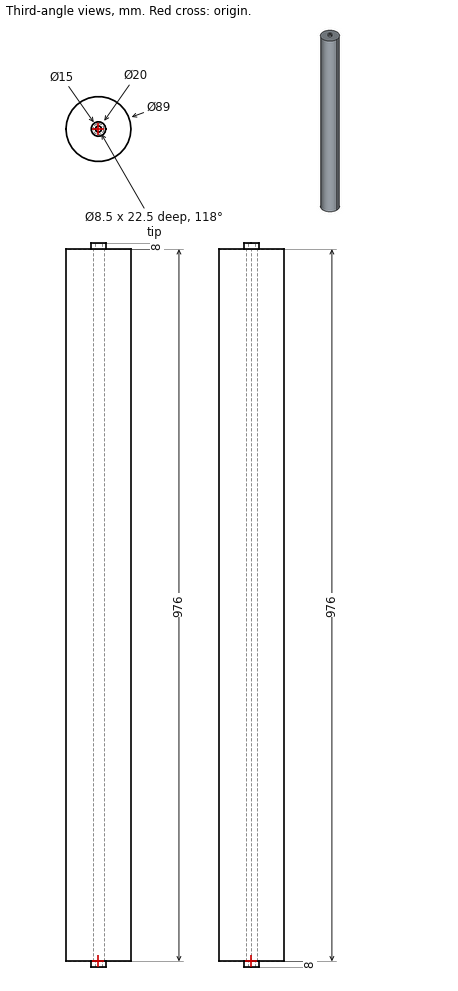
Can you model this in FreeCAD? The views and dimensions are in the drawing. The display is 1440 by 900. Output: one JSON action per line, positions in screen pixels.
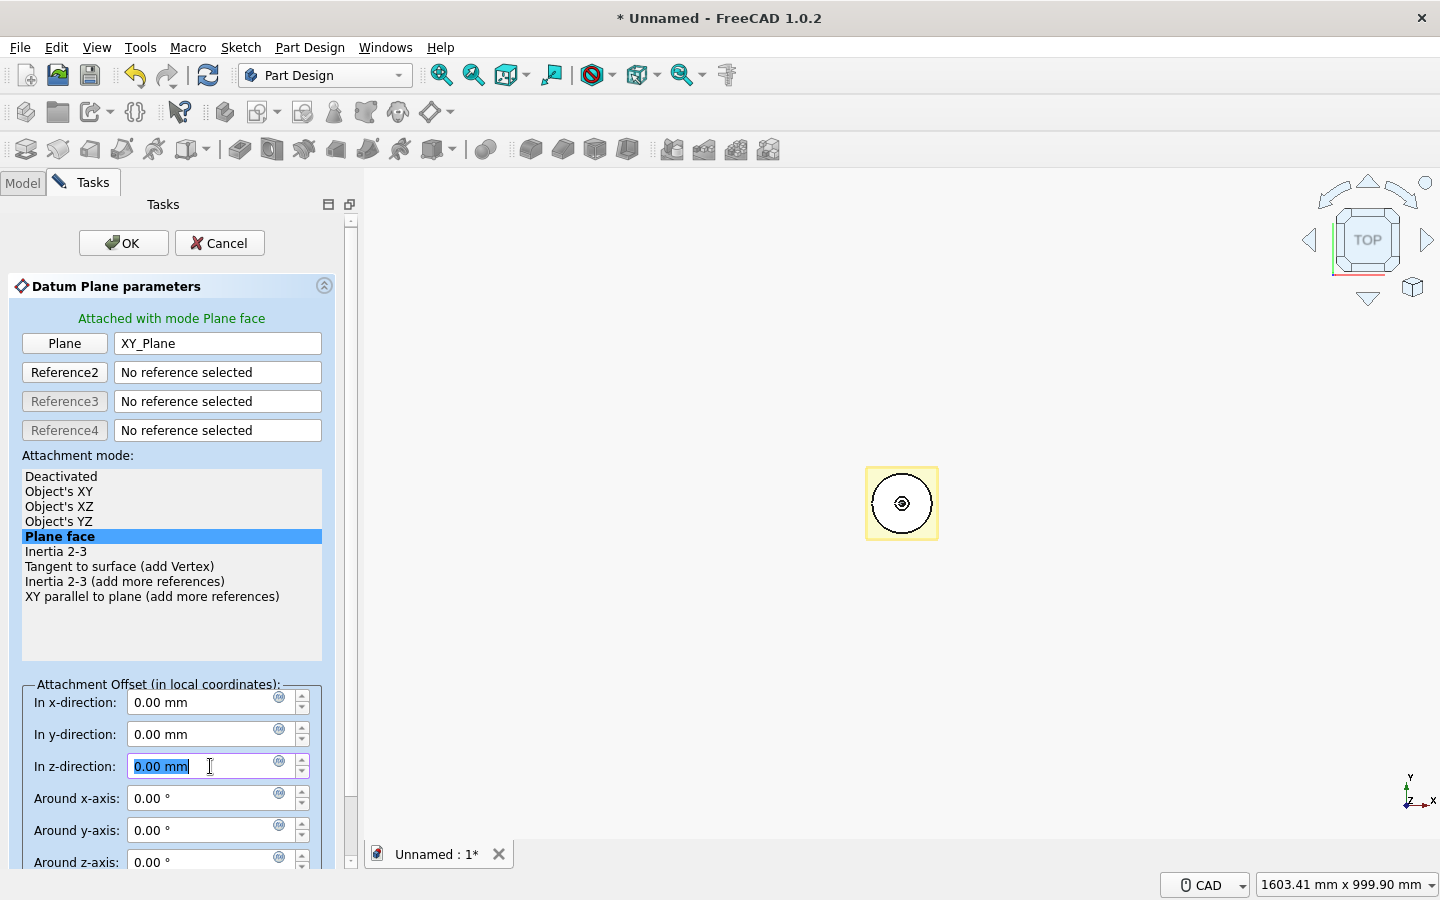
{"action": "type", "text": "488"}
{"action": "key", "text": "Tab"}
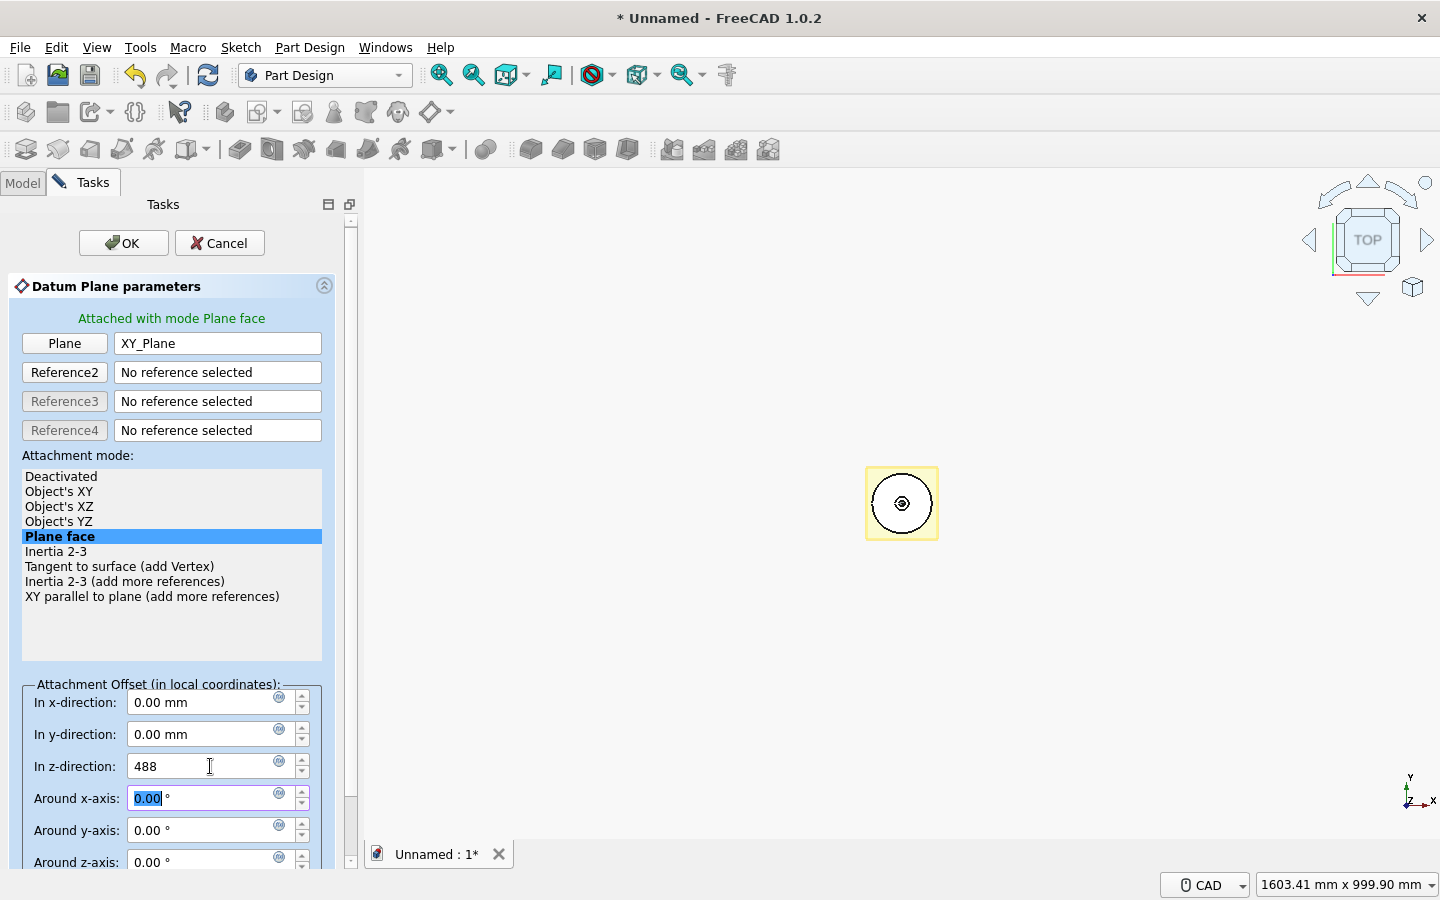
{"action": "left_click", "coordinate": [124, 243]}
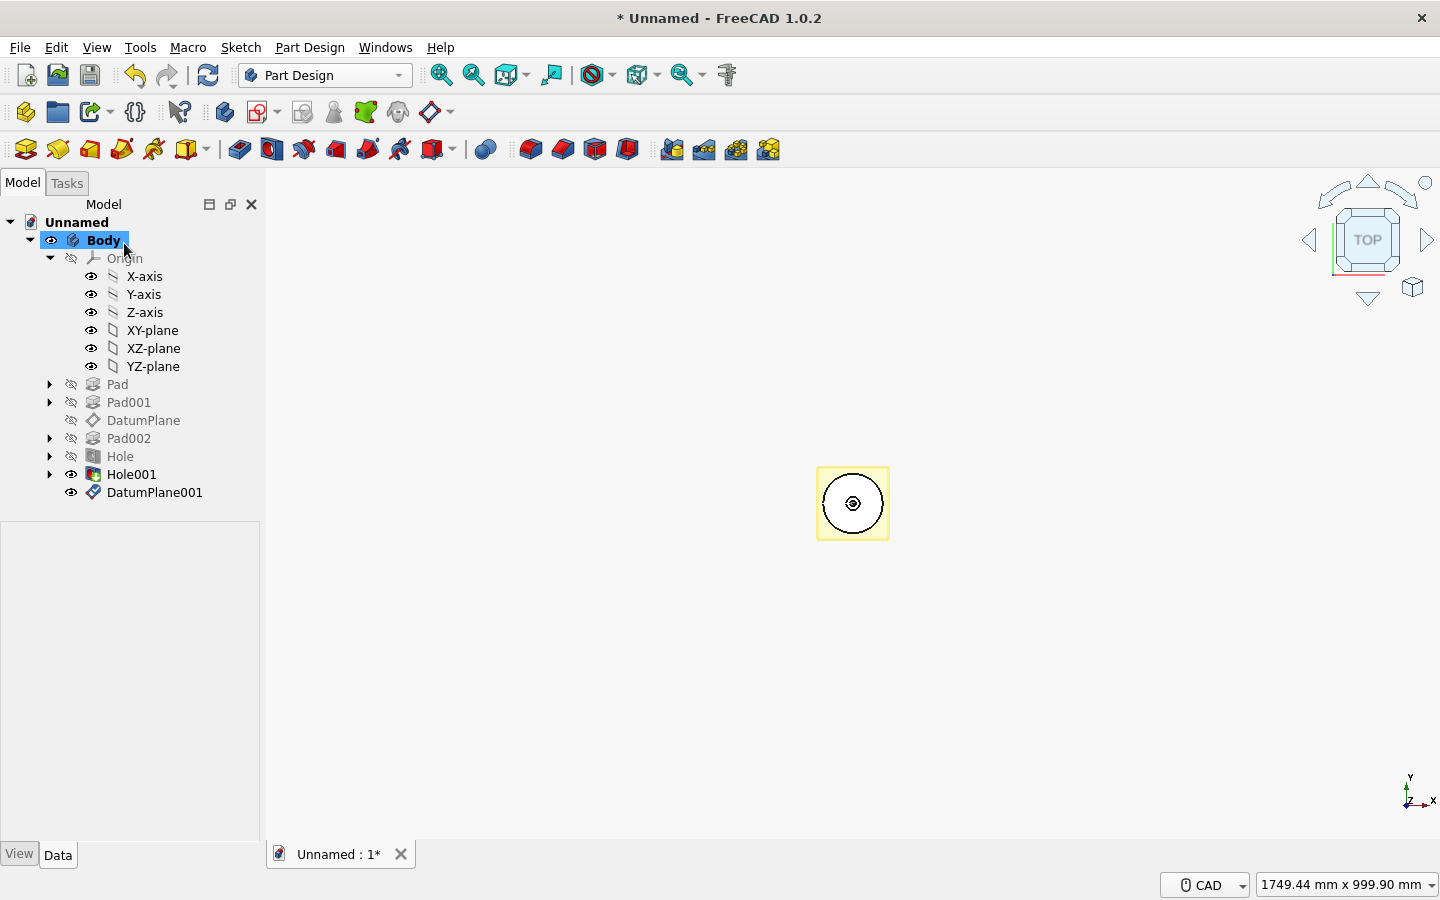
{"action": "left_click", "coordinate": [116, 492]}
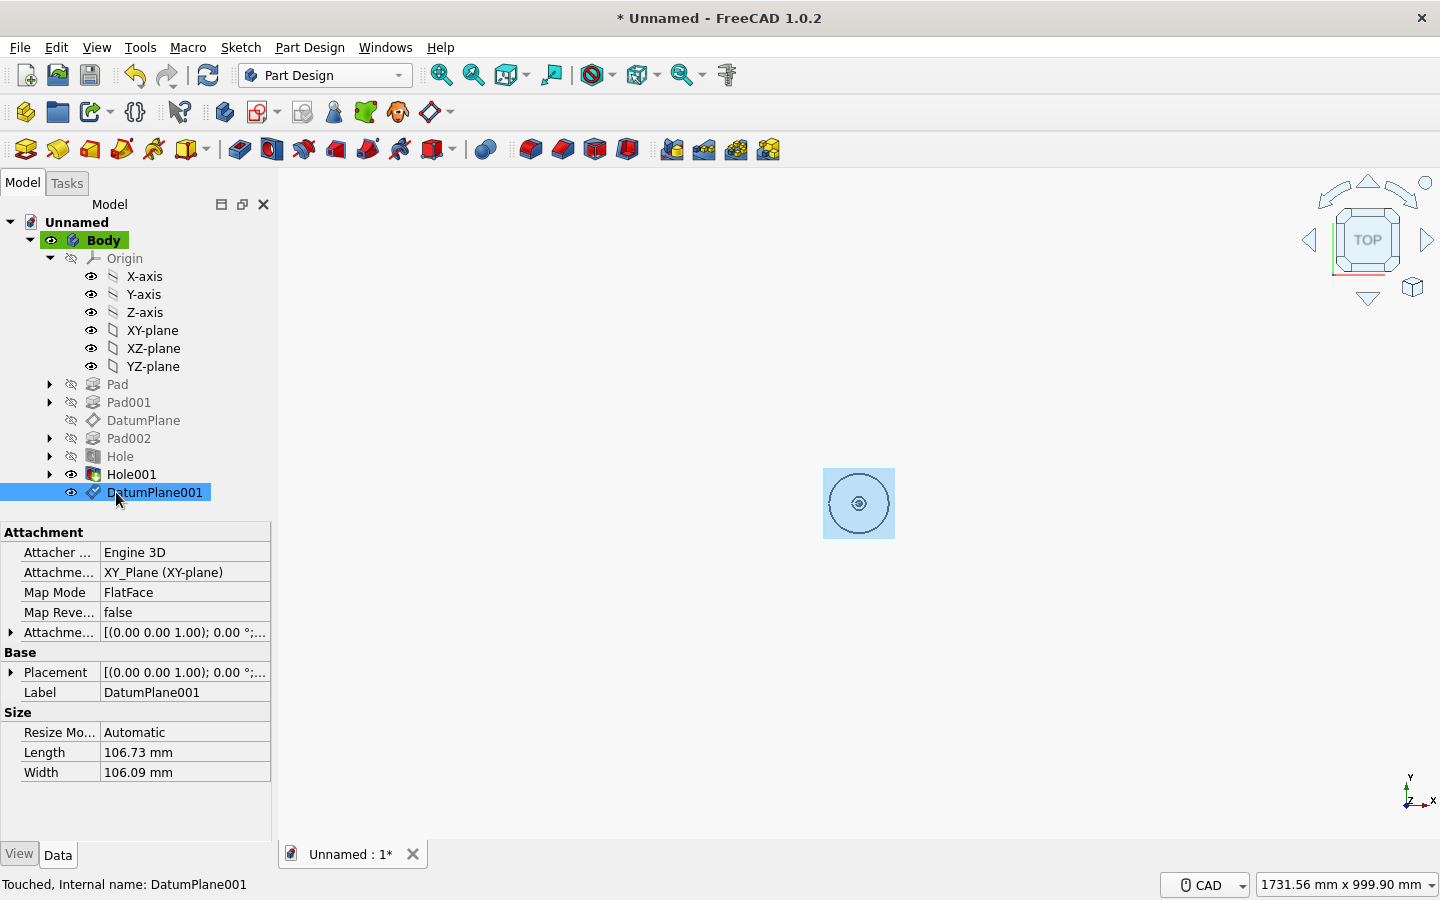
{"action": "left_click", "coordinate": [258, 112]}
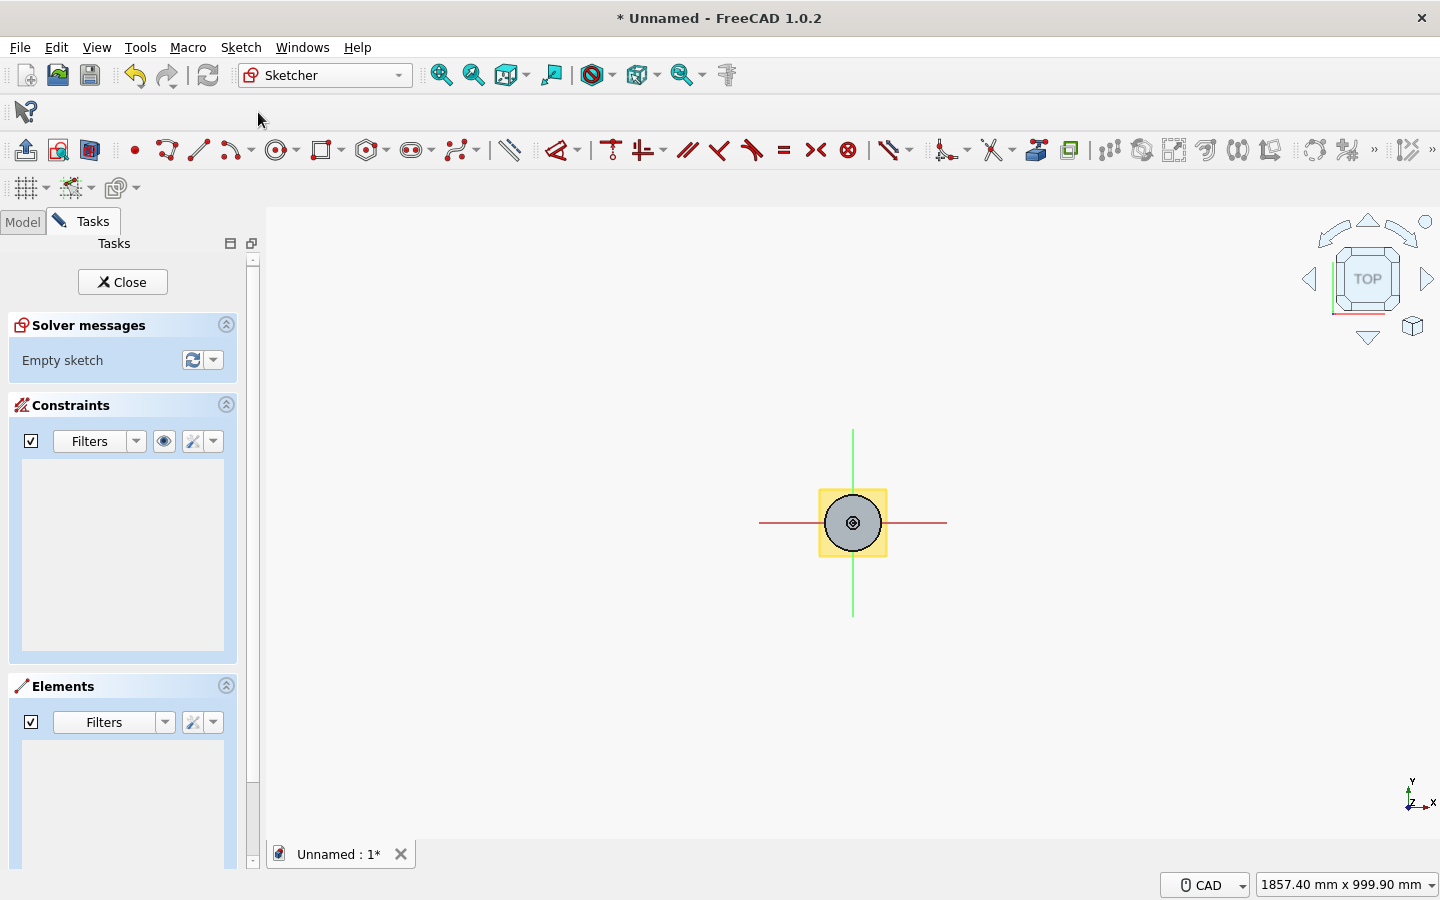
{"action": "left_click", "coordinate": [90, 150]}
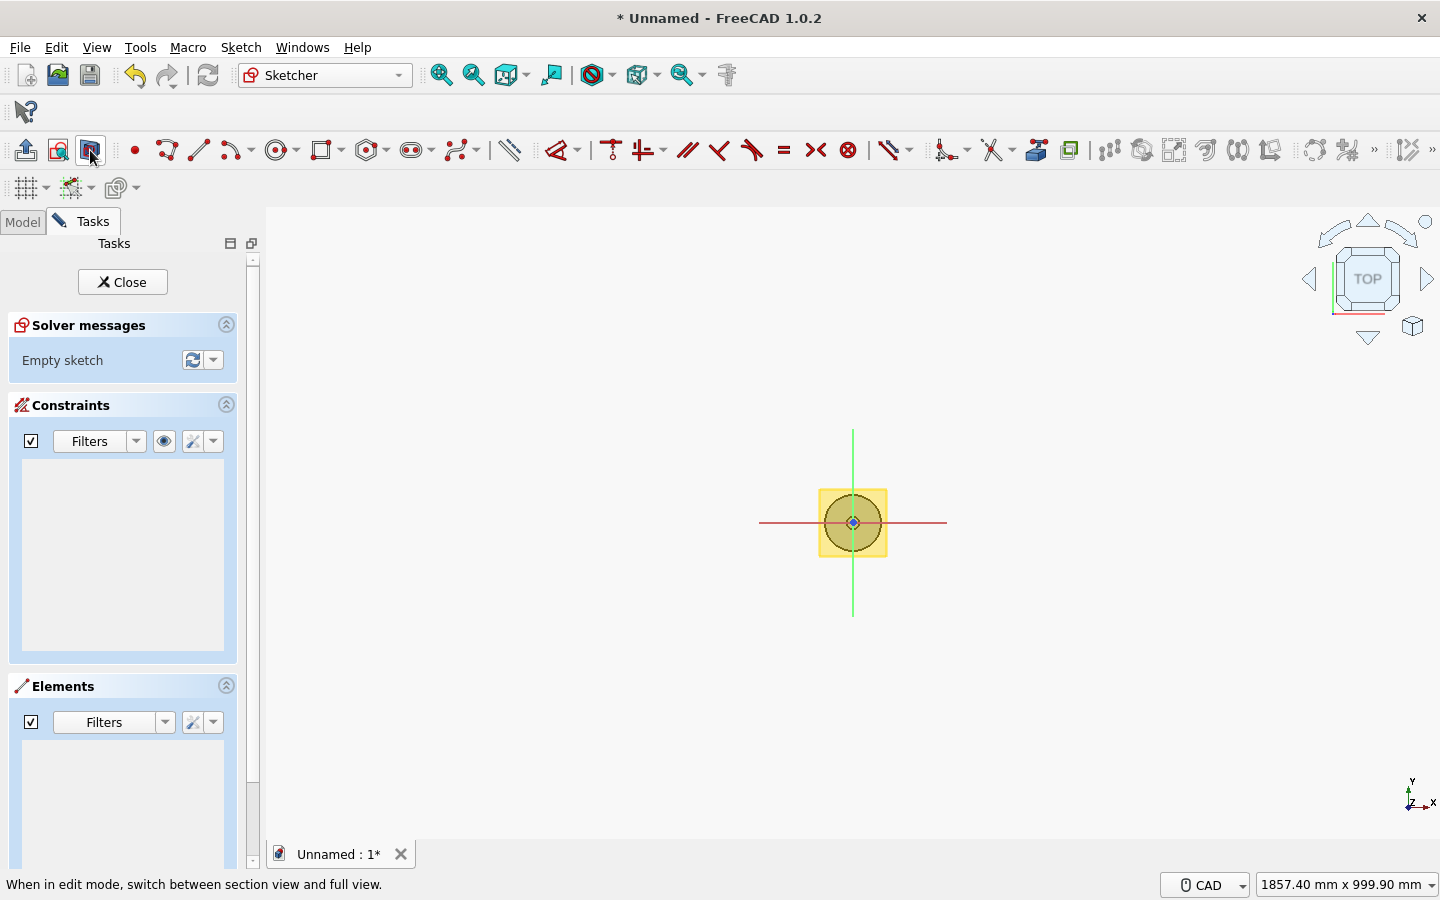
{"action": "scroll", "coordinate": [857, 523], "scroll_direction": "up", "scroll_amount": 15}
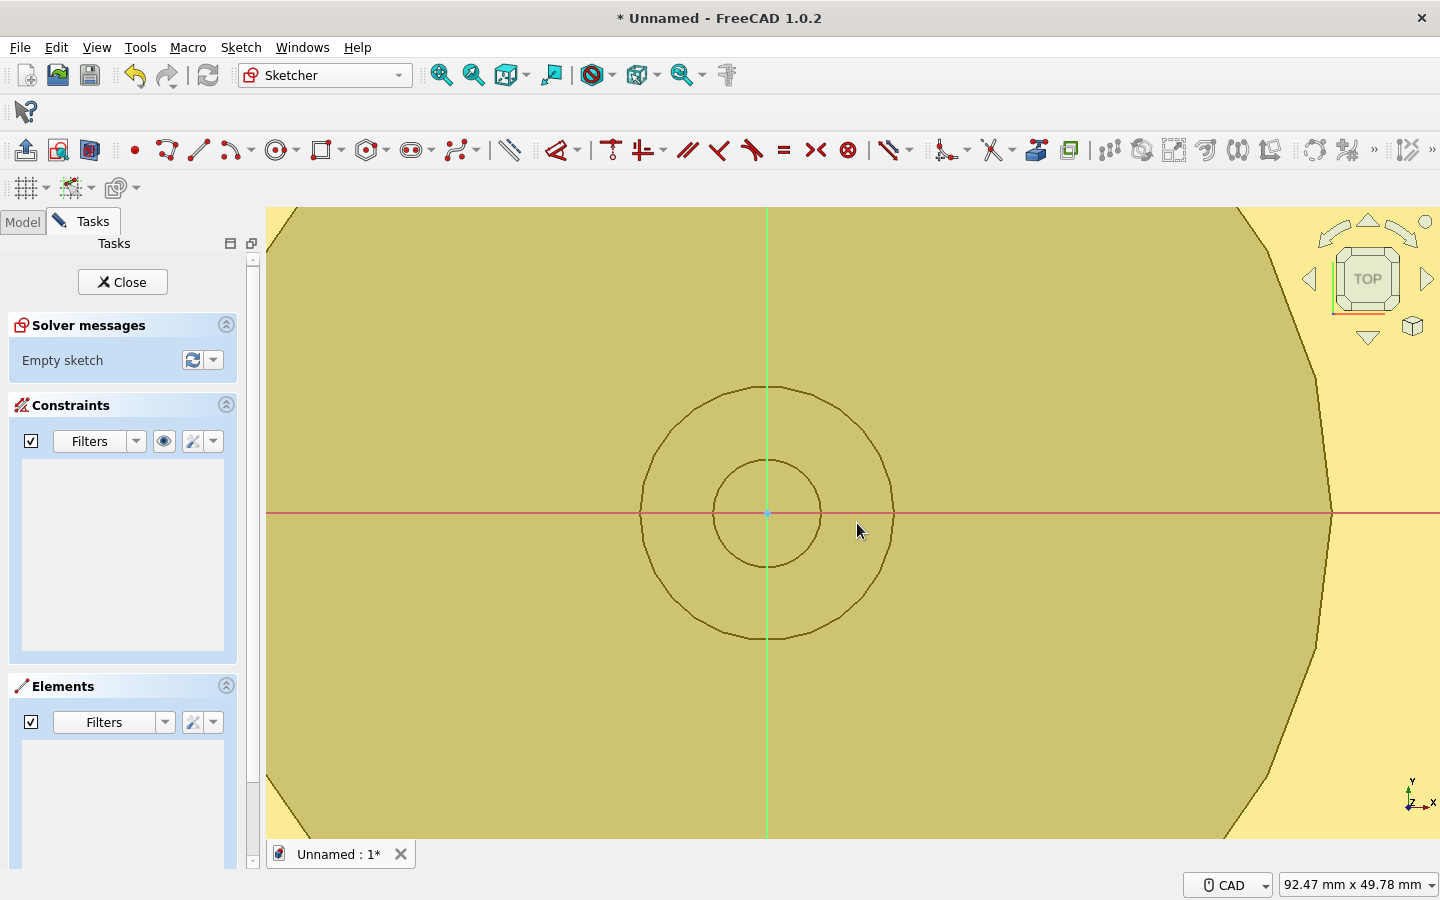
{"action": "scroll", "coordinate": [753, 506], "scroll_direction": "up", "scroll_amount": 4}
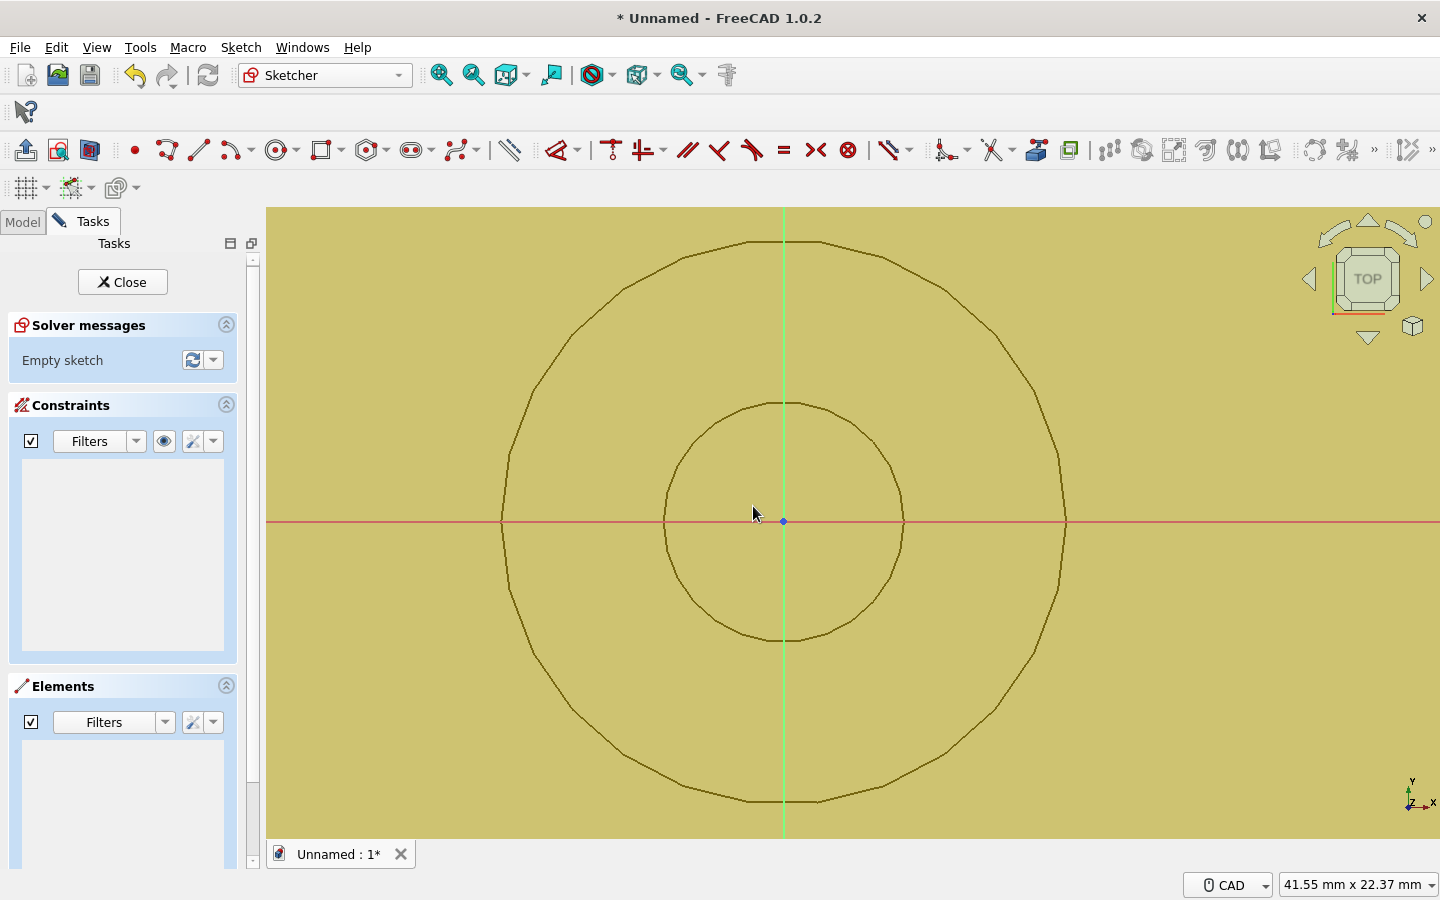
{"action": "left_click", "coordinate": [276, 150]}